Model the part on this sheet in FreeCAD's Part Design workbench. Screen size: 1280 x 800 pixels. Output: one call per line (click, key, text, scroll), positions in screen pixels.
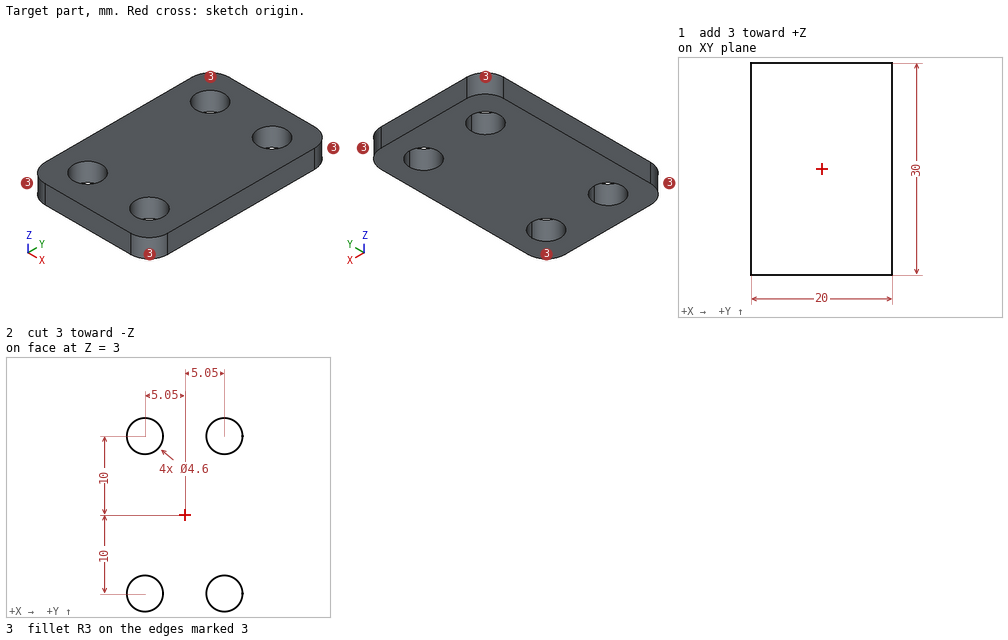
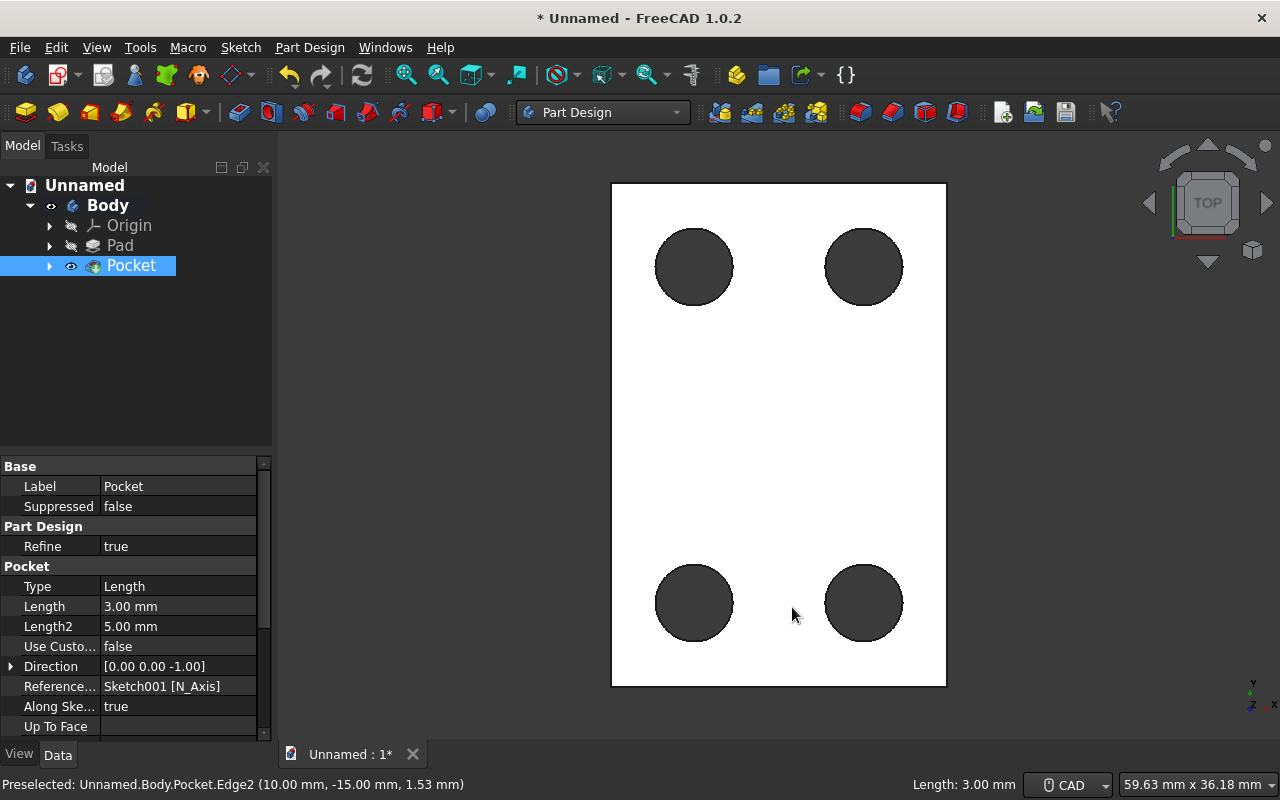
key(1)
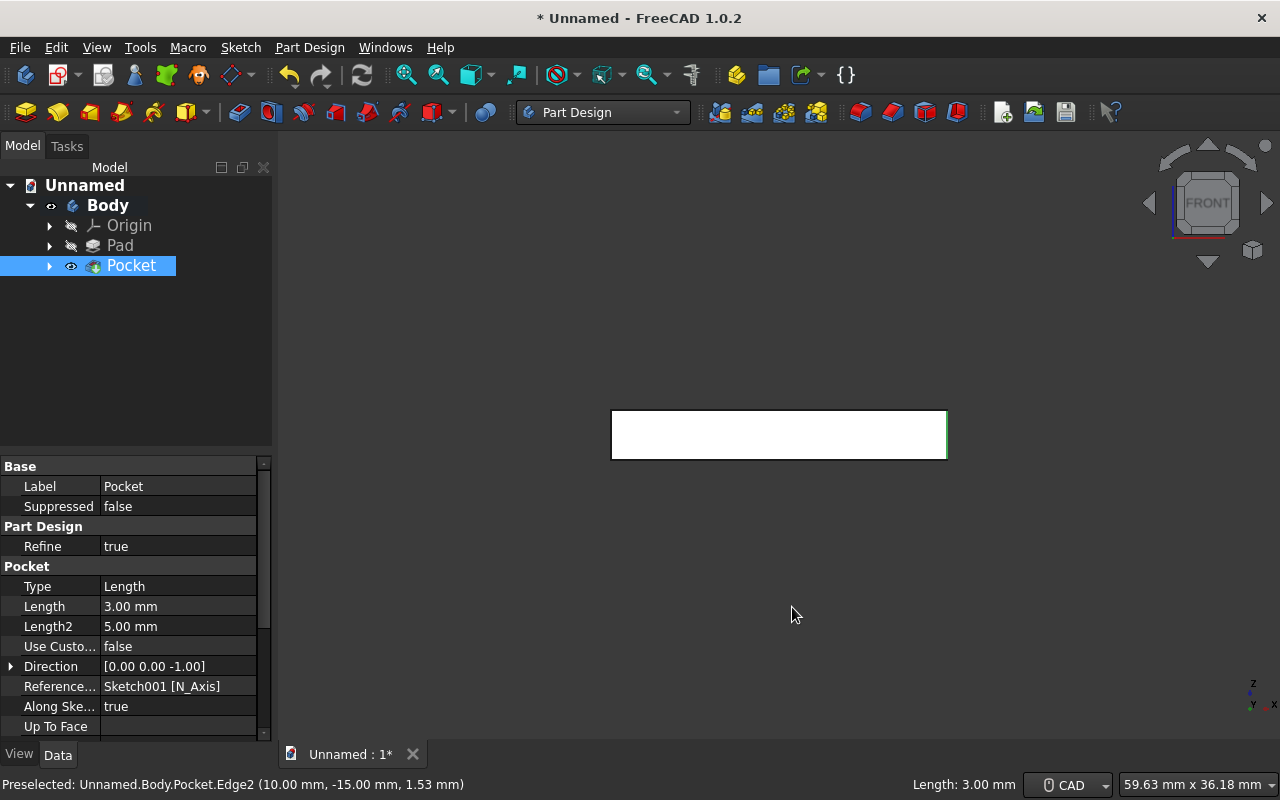
key(v)
key(f)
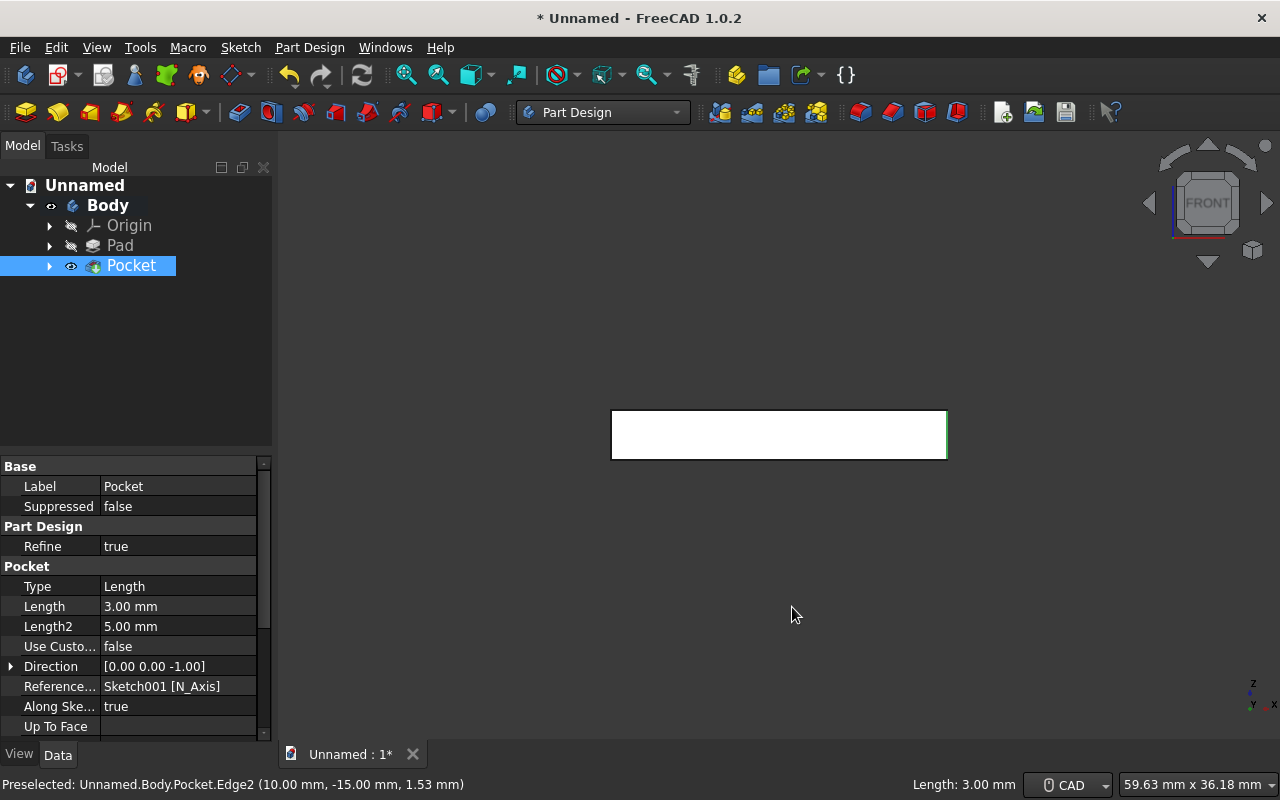
click(611, 434, ctrl)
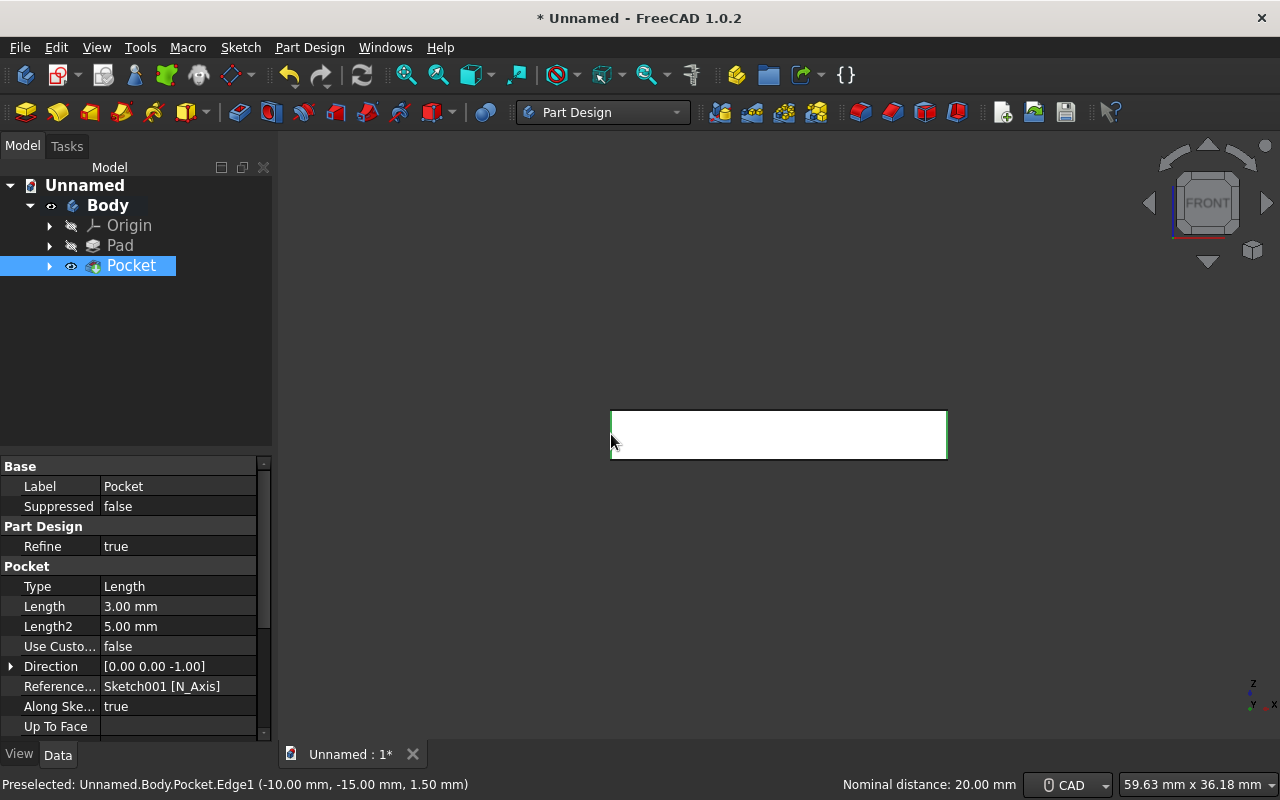
key(3)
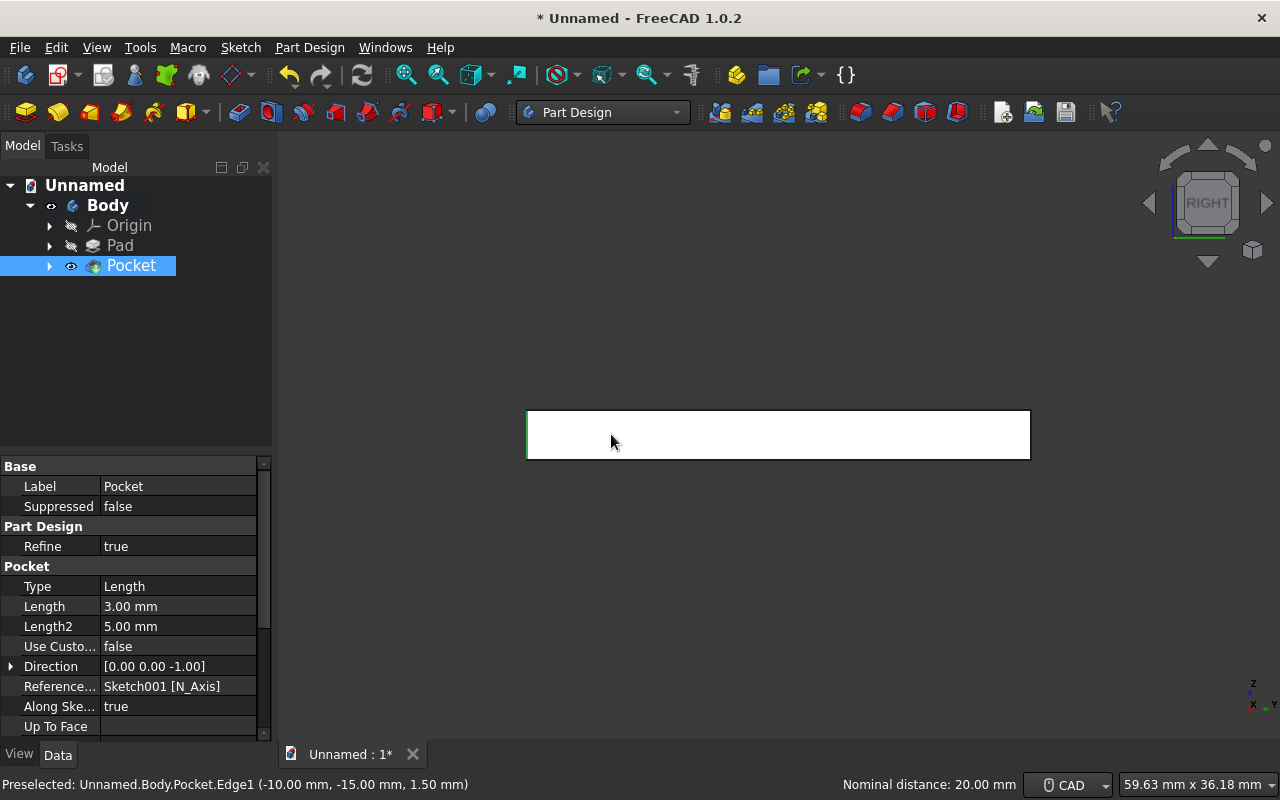
click(1031, 434, ctrl)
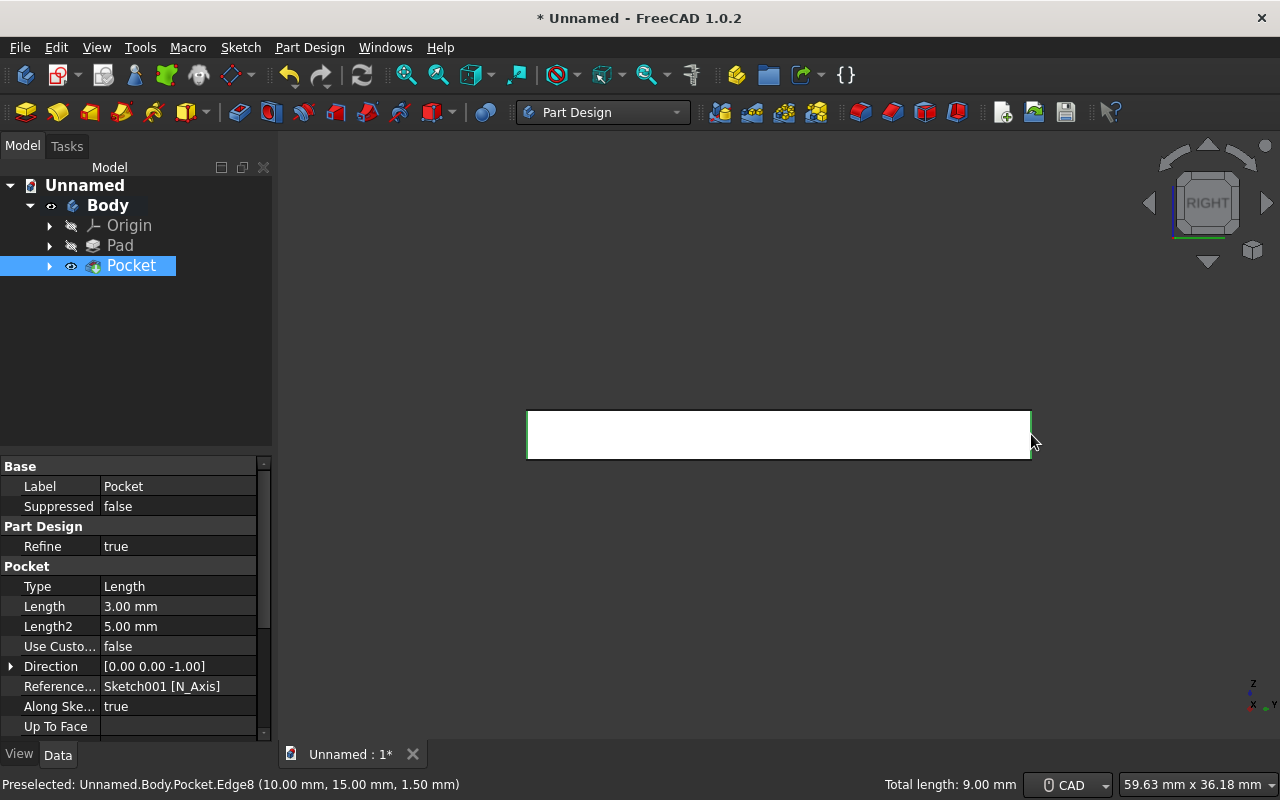
key(5)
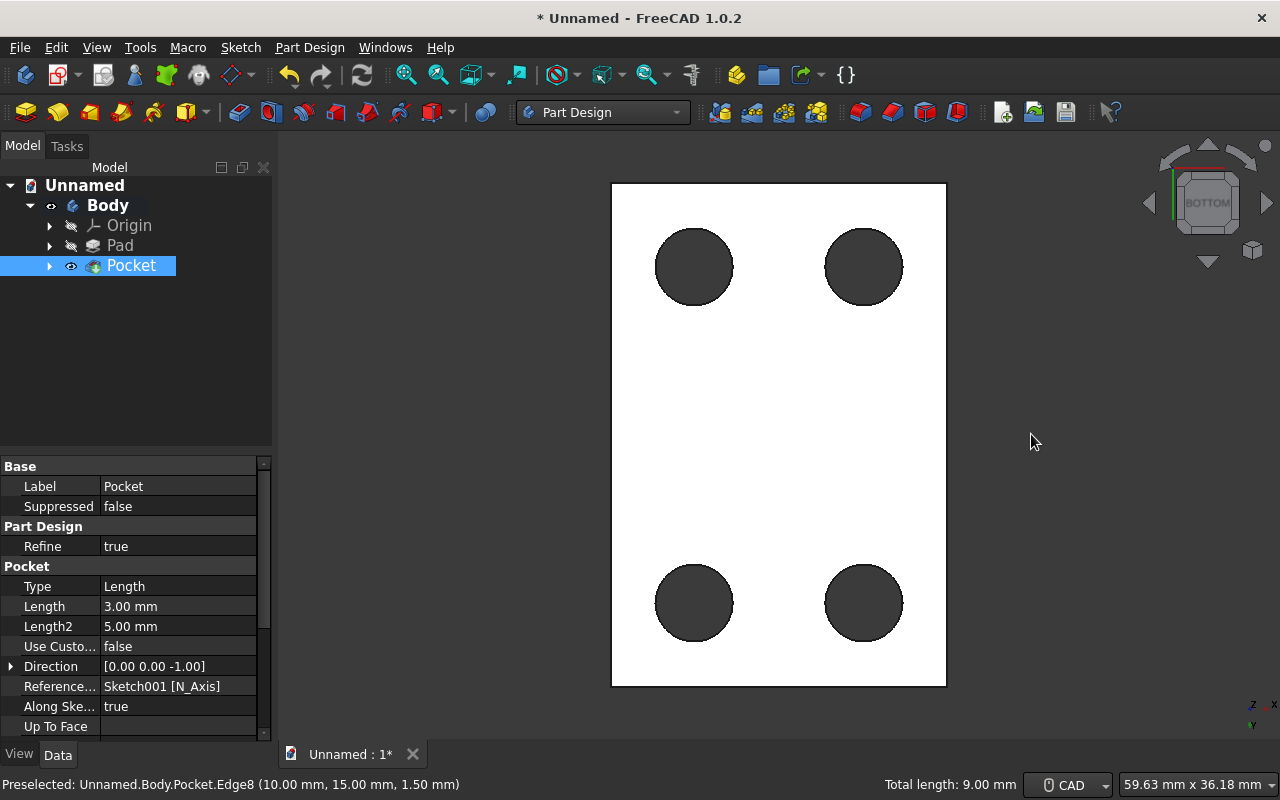
key(4)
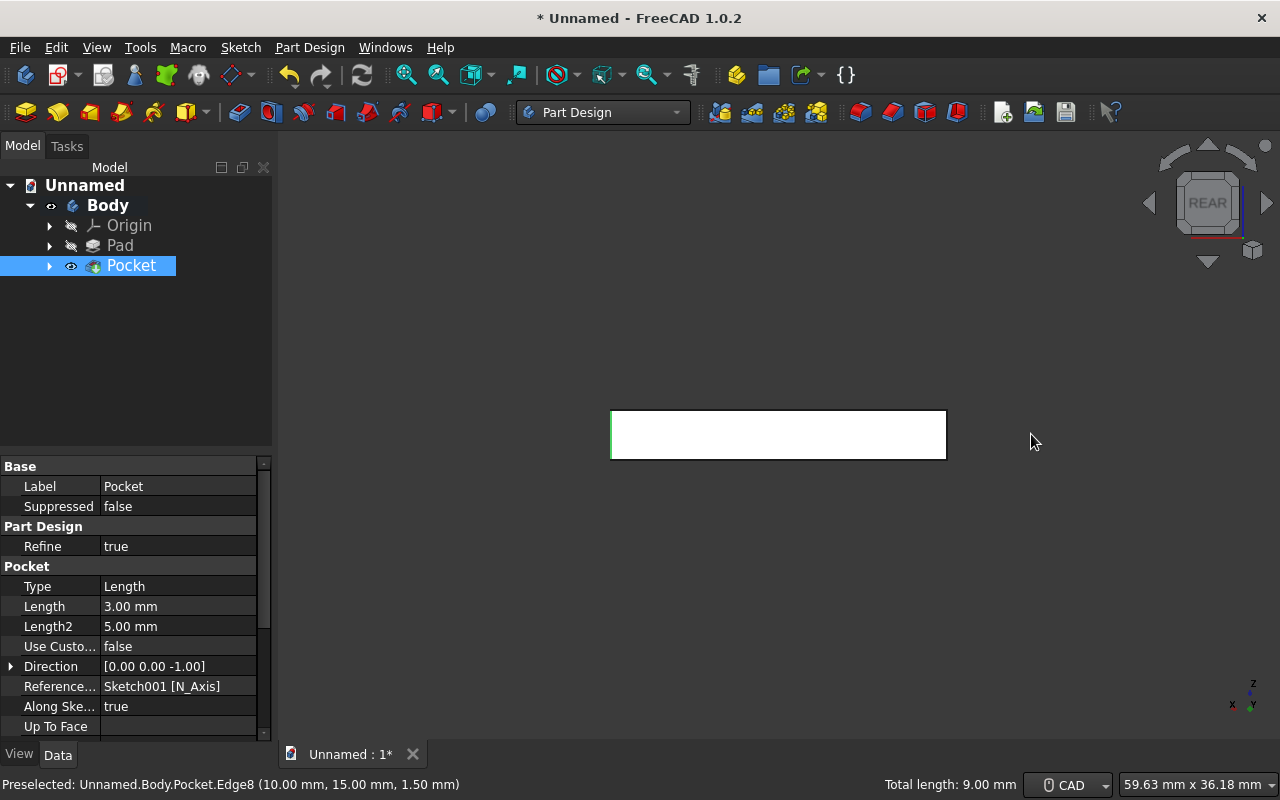
click(408, 76)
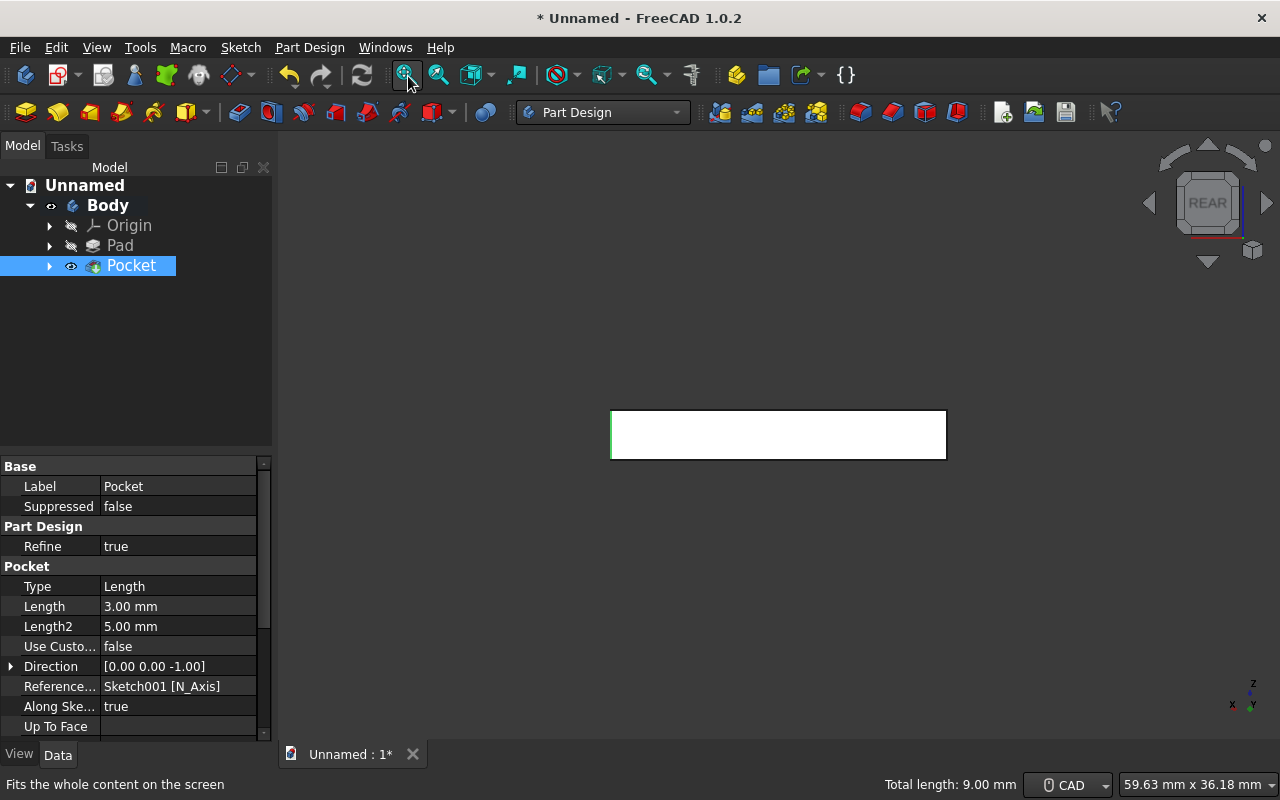
click(947, 434, ctrl)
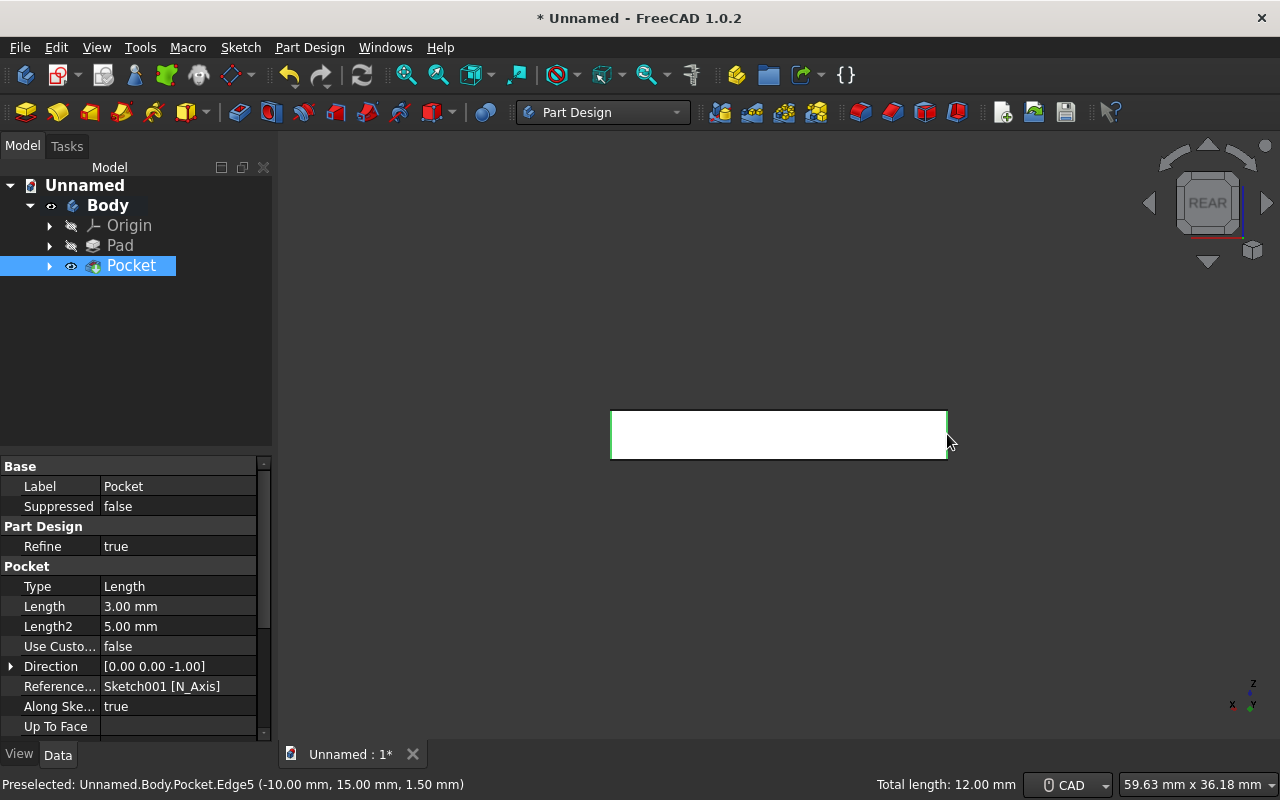
click(862, 112)